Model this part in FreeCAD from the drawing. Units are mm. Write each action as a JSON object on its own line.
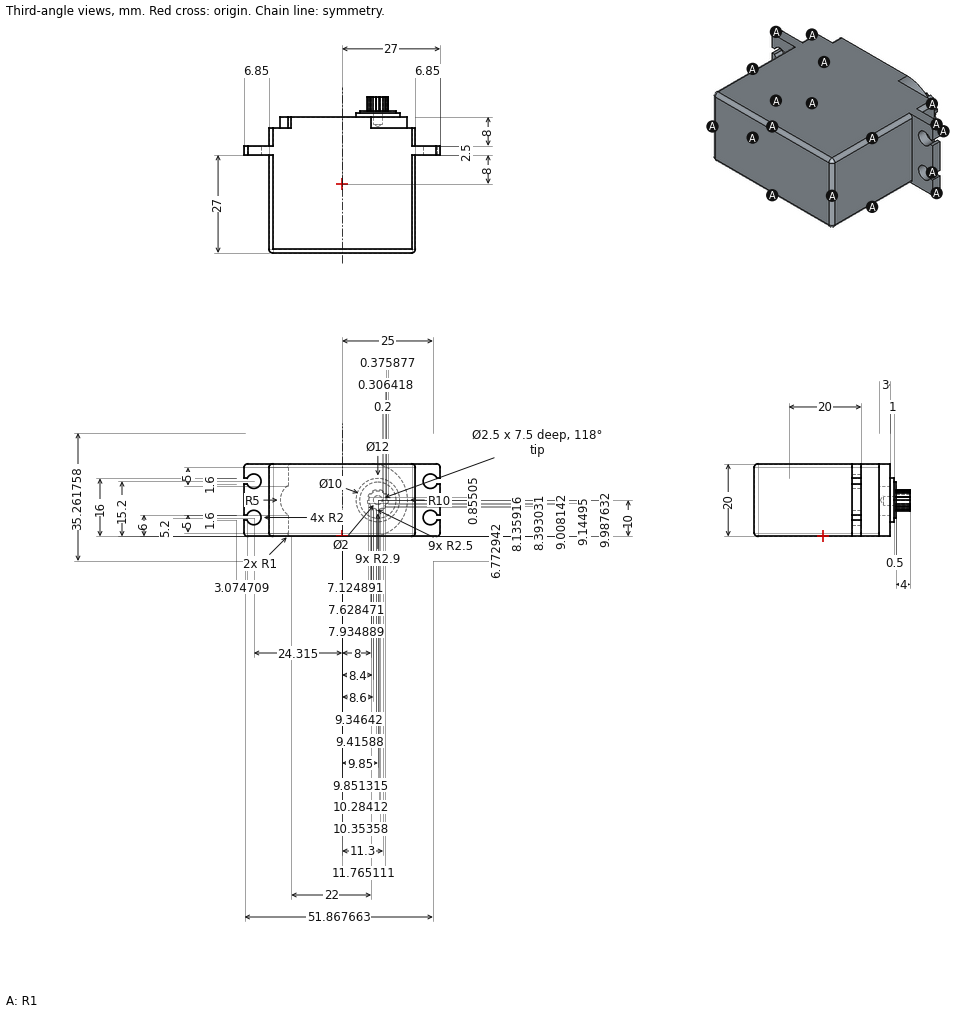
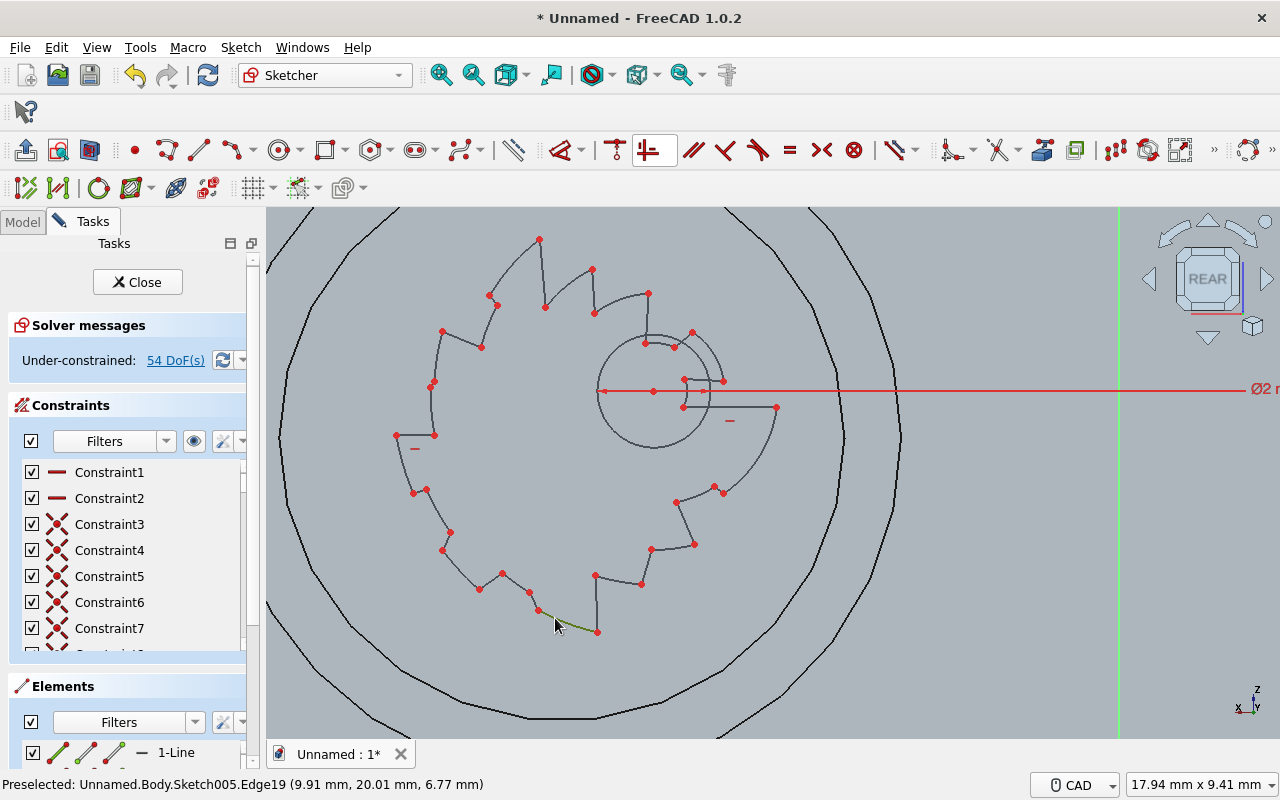
{"action": "left_click", "coordinate": [665, 550]}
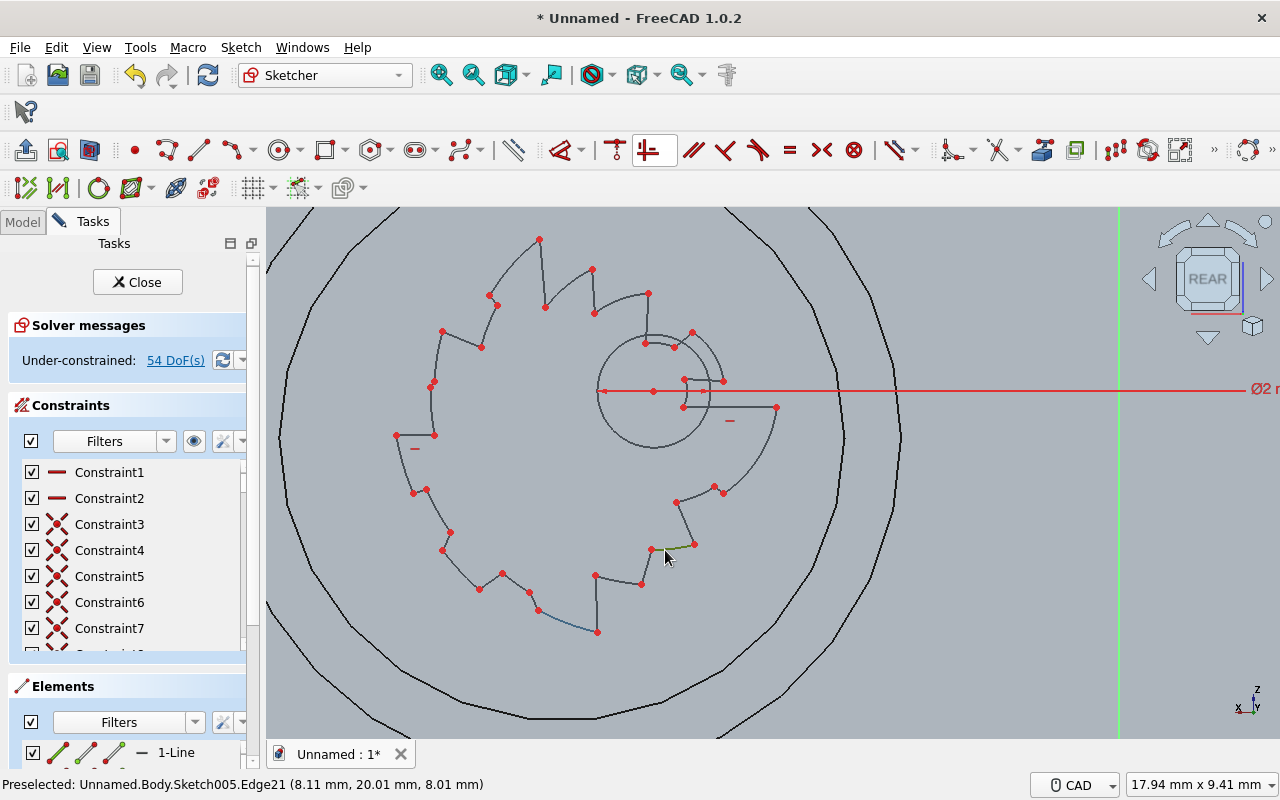
{"action": "left_click", "coordinate": [747, 473]}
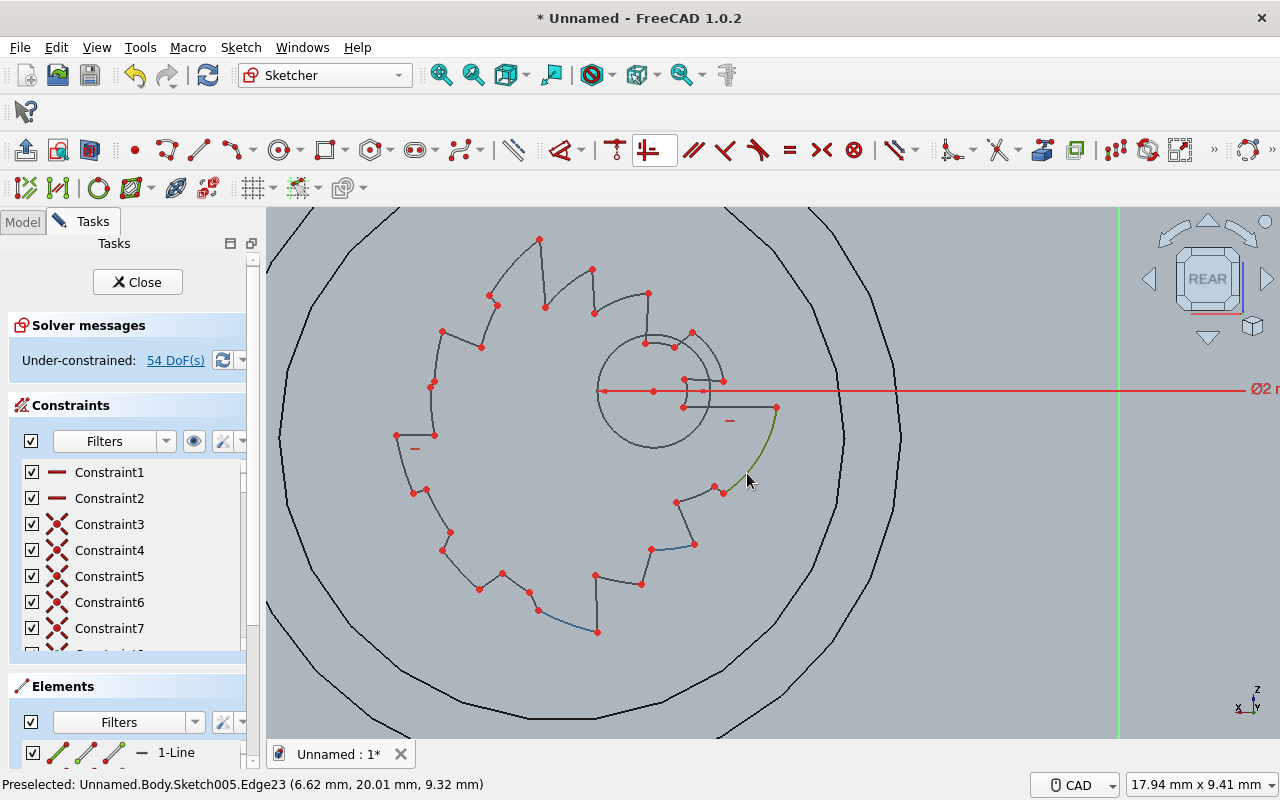
{"action": "left_click", "coordinate": [719, 364]}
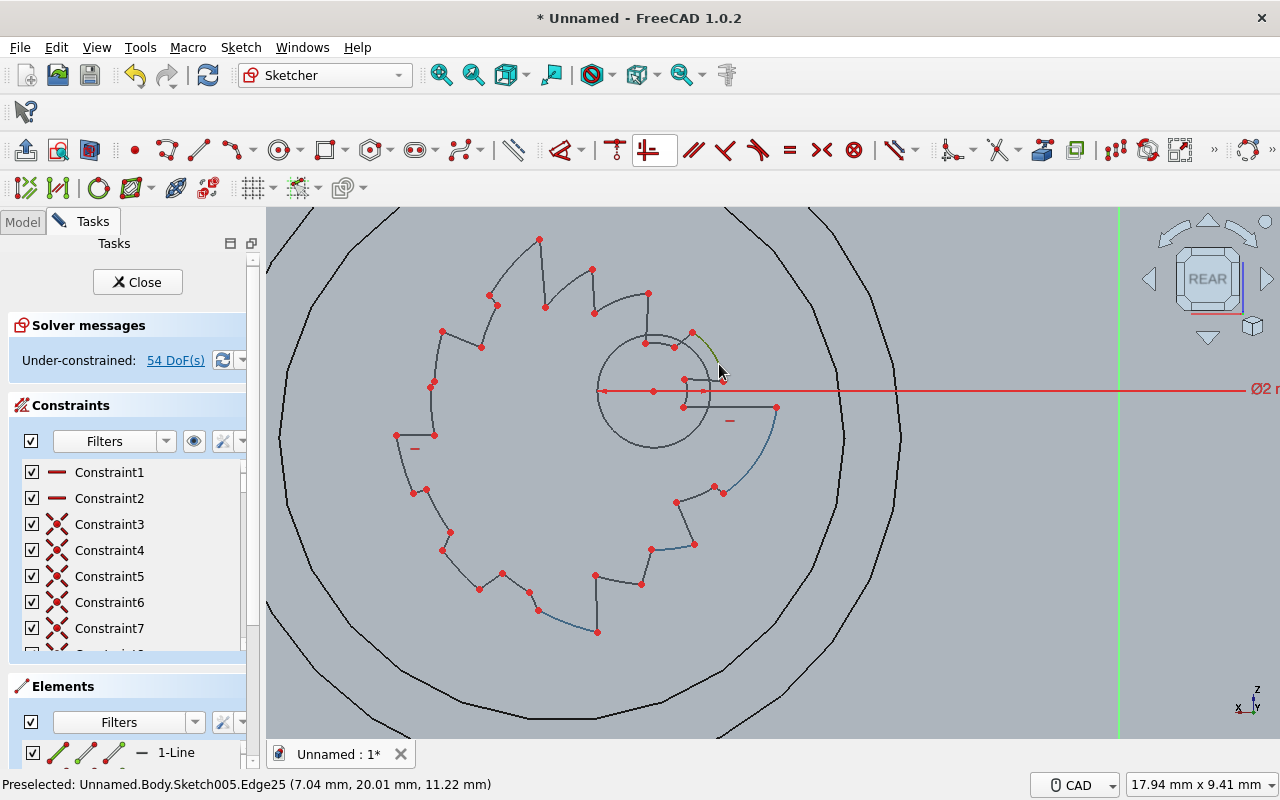
{"action": "left_click", "coordinate": [631, 296]}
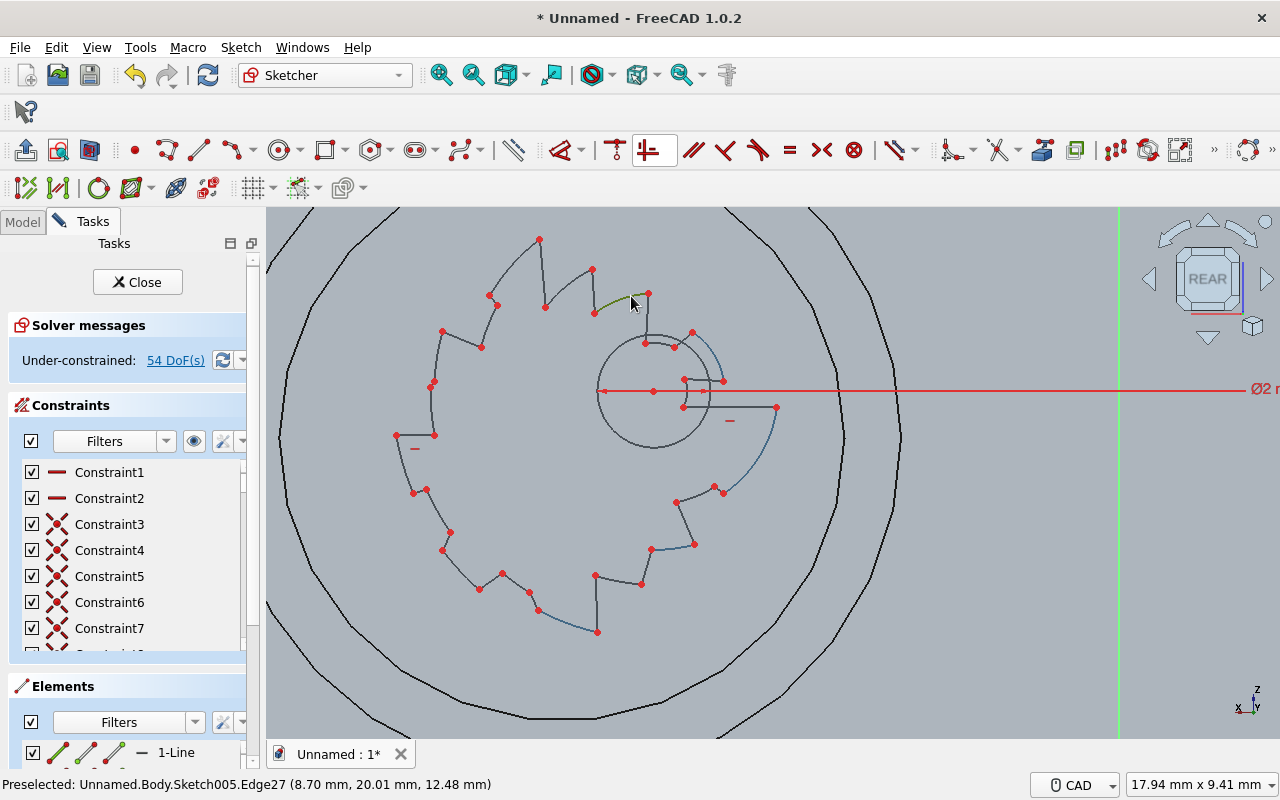
{"action": "left_click", "coordinate": [523, 254]}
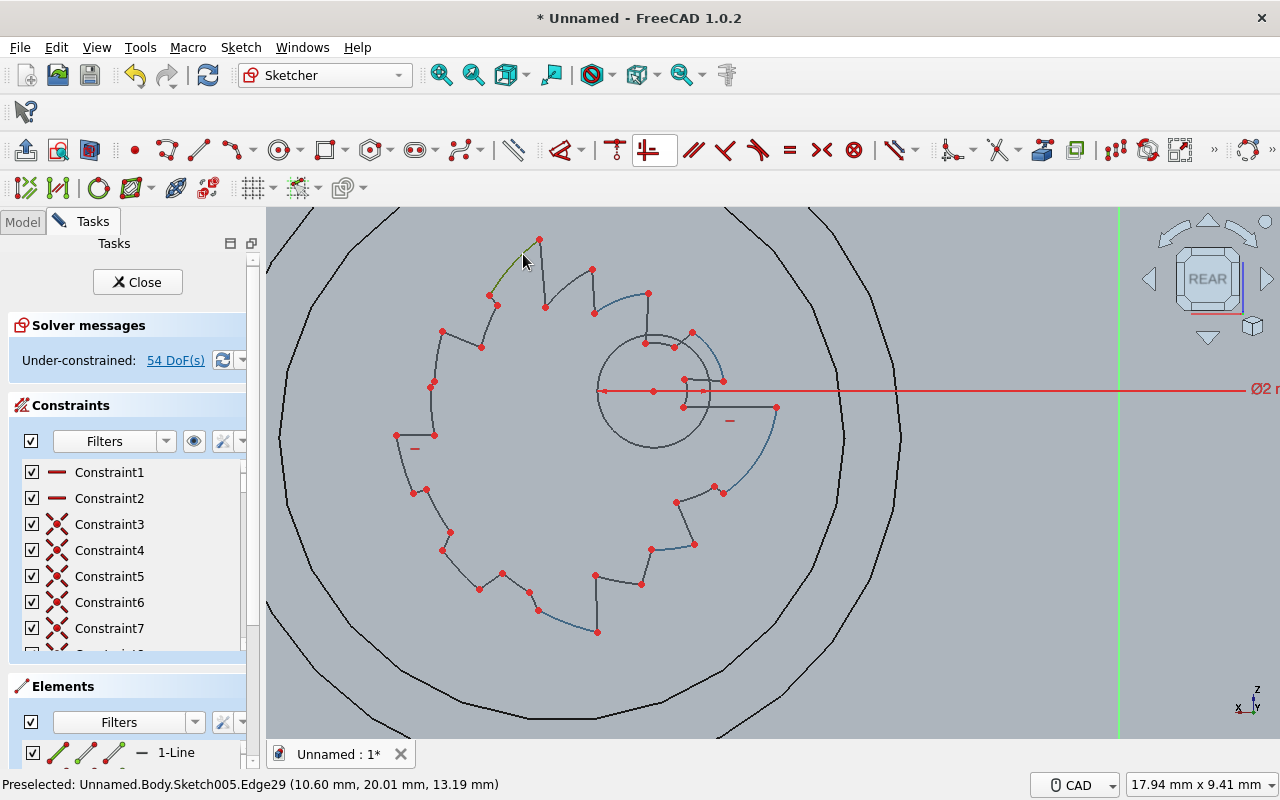
{"action": "left_click", "coordinate": [439, 347]}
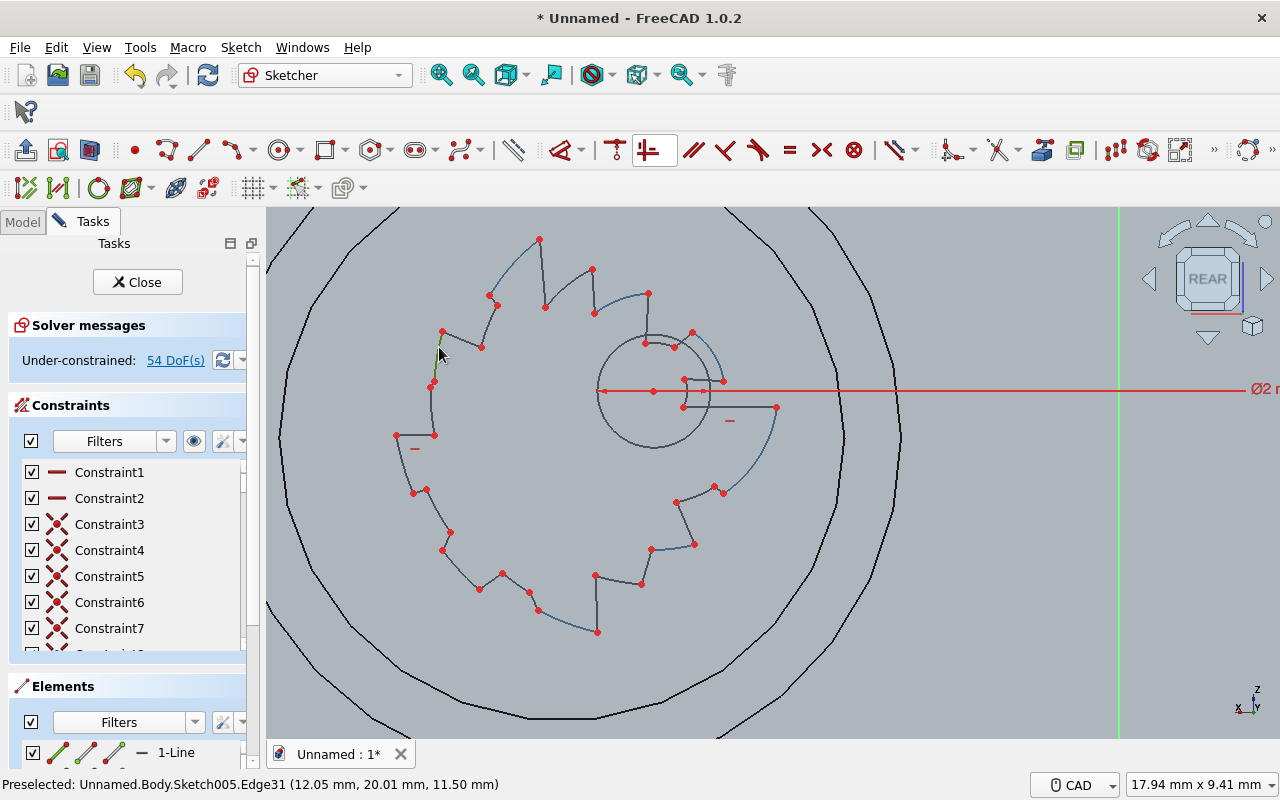
{"action": "left_click", "coordinate": [400, 453]}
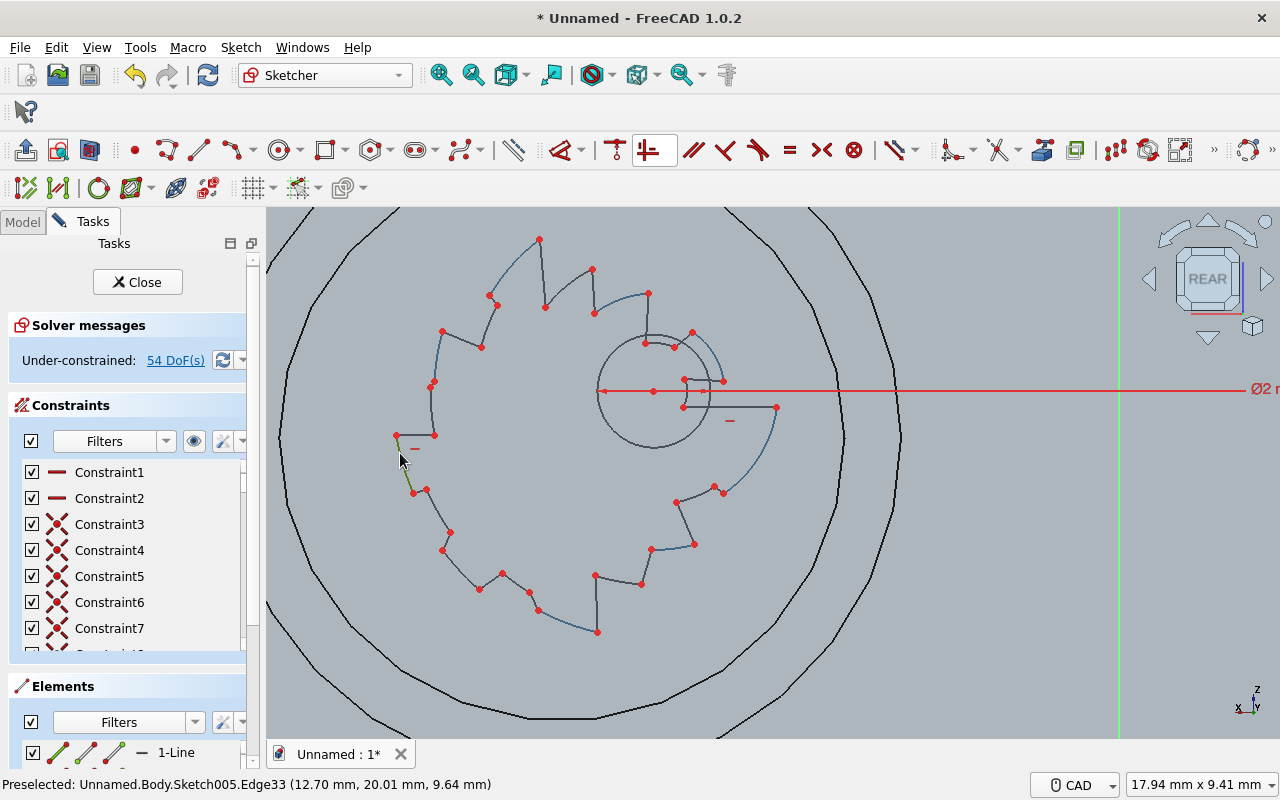
{"action": "left_click", "coordinate": [453, 563]}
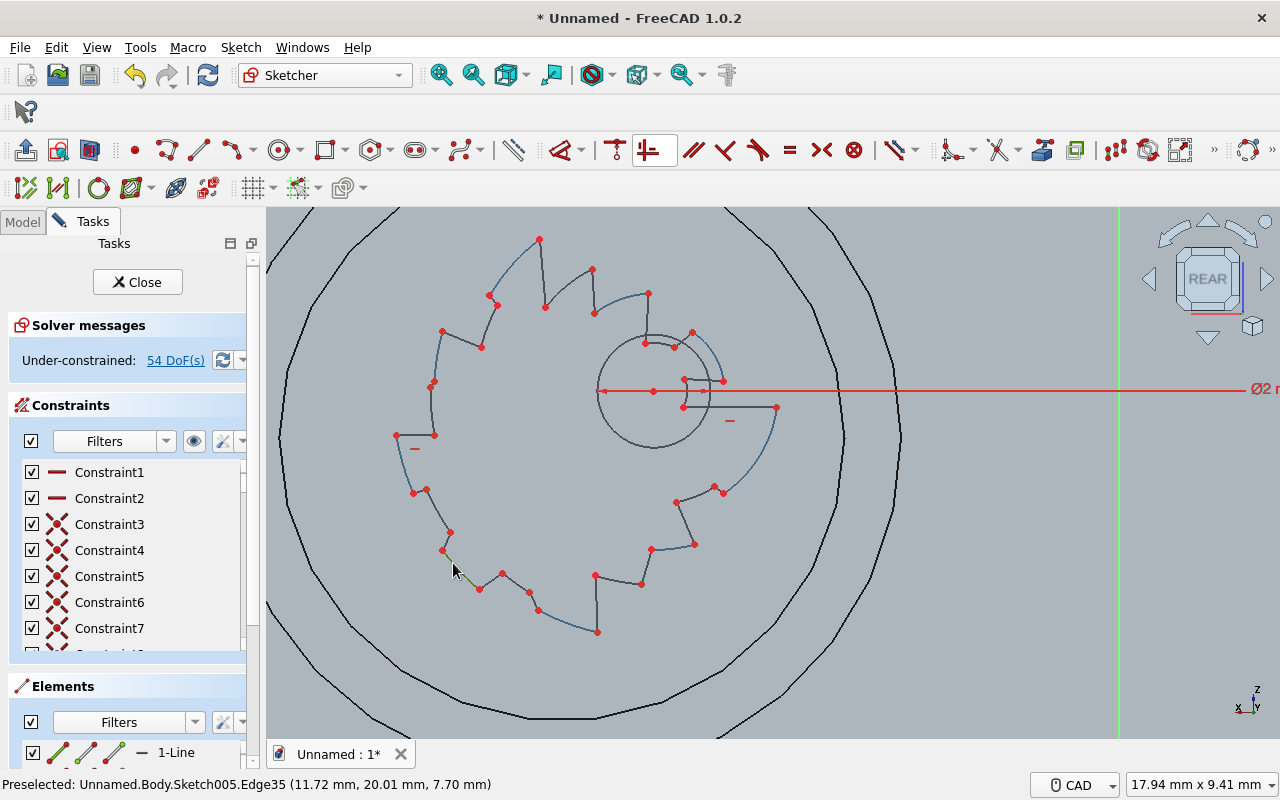
{"action": "left_click", "coordinate": [790, 150]}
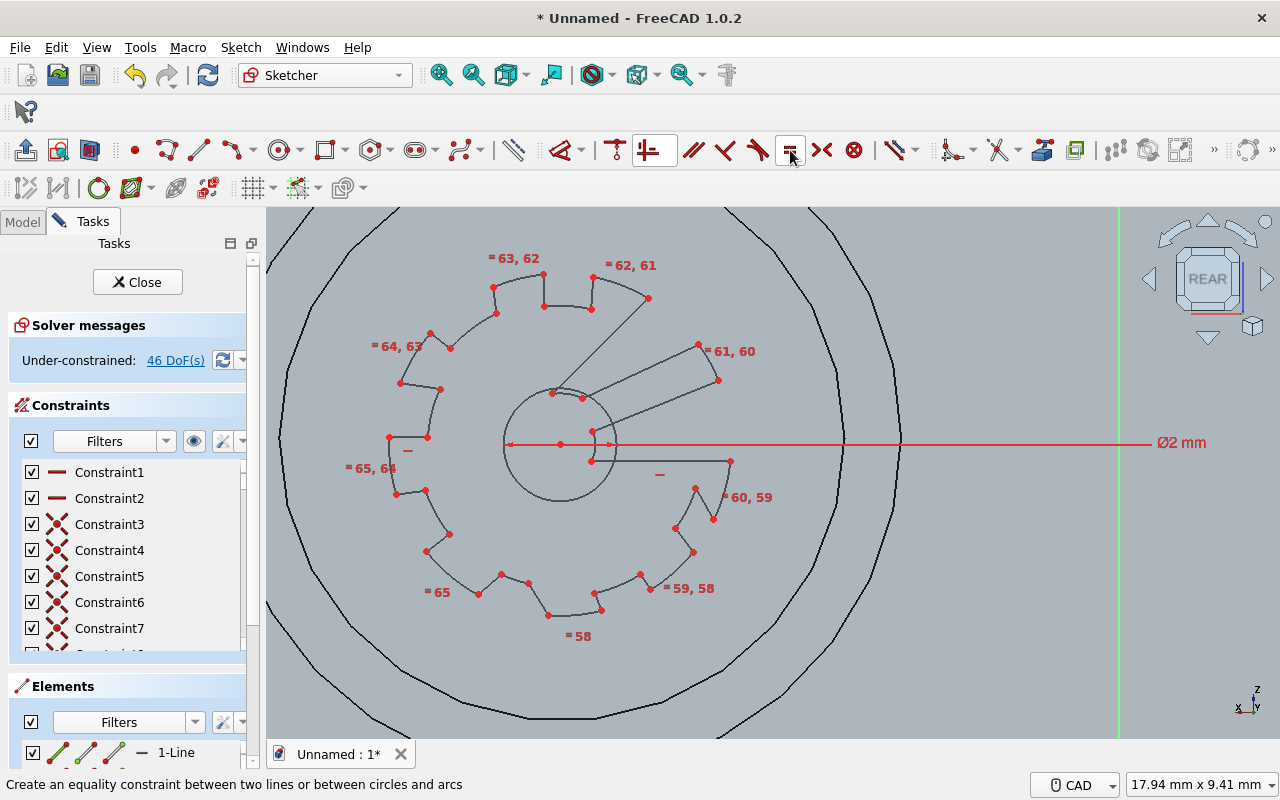
{"action": "left_click", "coordinate": [609, 589]}